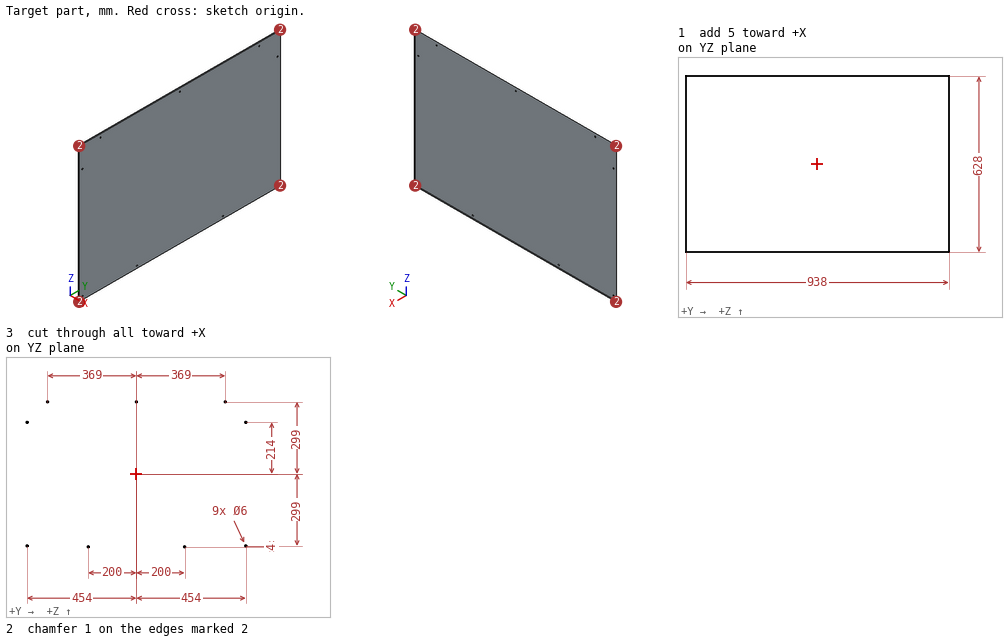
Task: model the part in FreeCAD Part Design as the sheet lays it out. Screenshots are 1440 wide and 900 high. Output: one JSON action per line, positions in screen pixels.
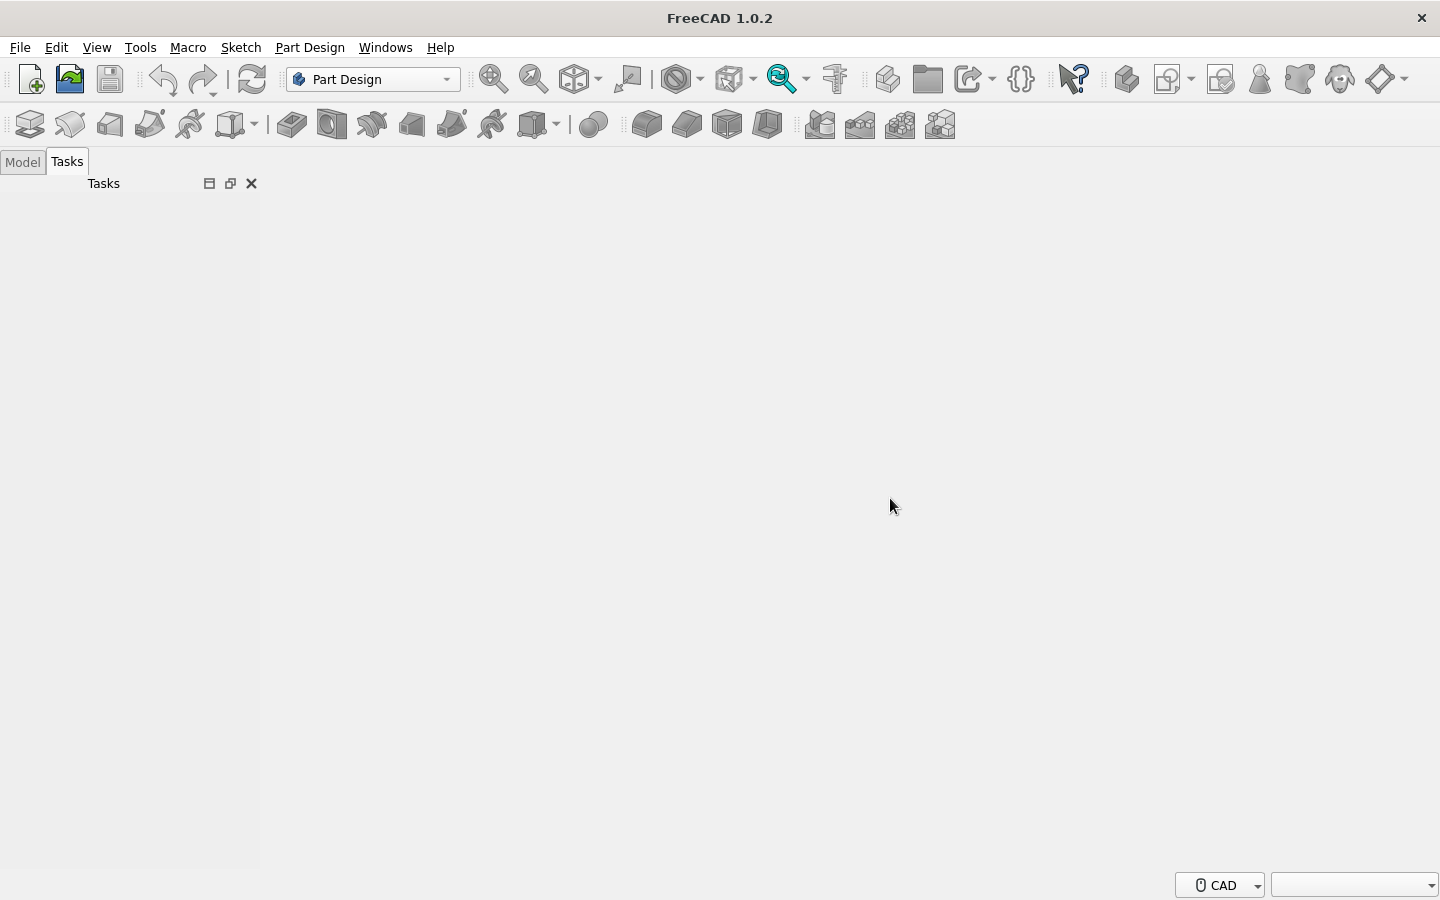
{"action": "key", "text": "ctrl+n"}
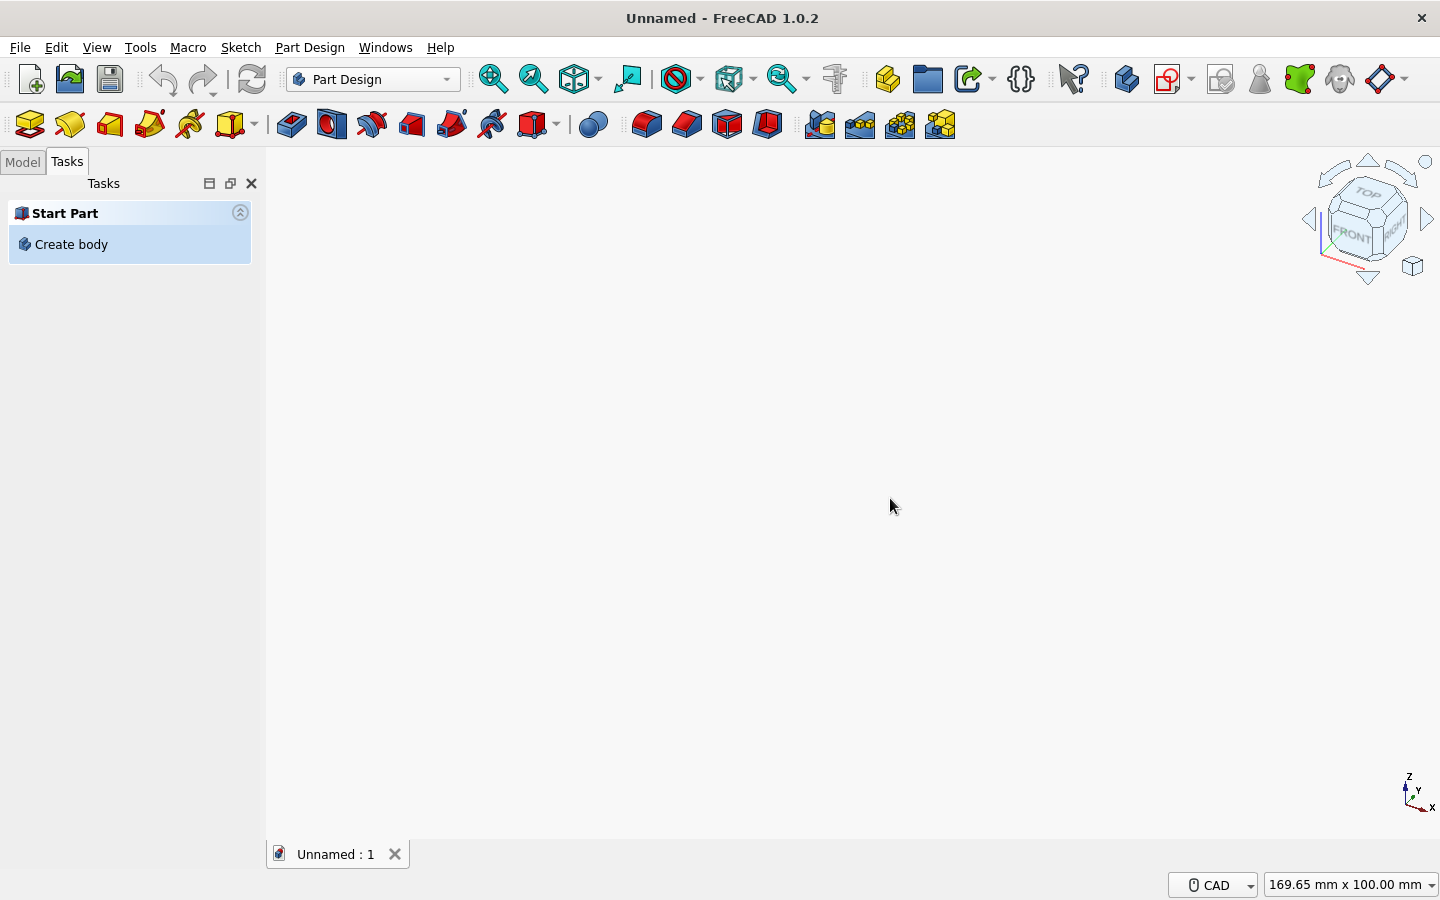
{"action": "left_click", "coordinate": [1168, 80]}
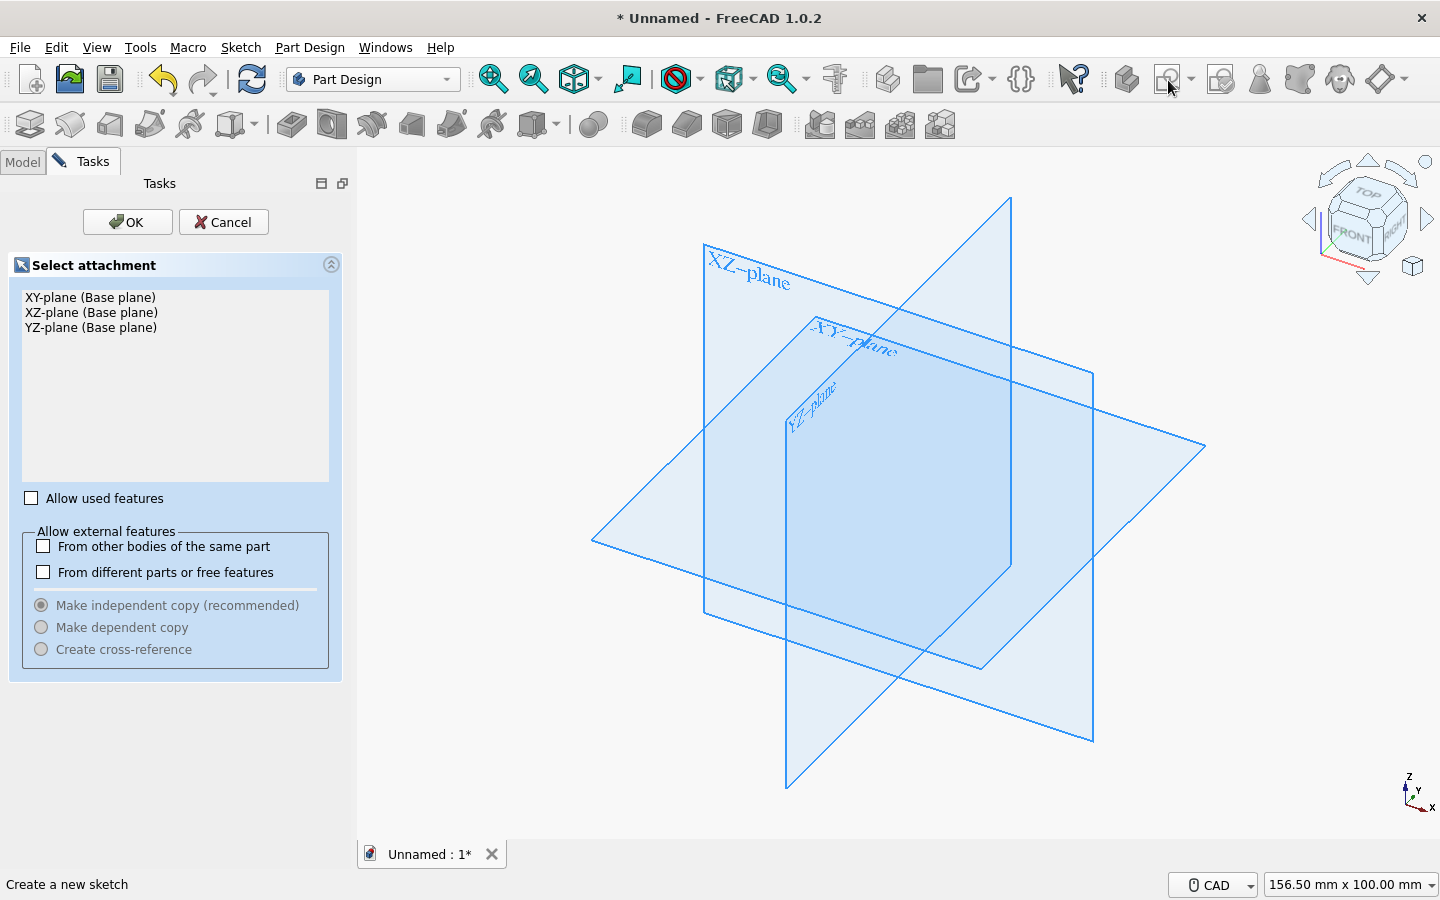
{"action": "left_click", "coordinate": [82, 328]}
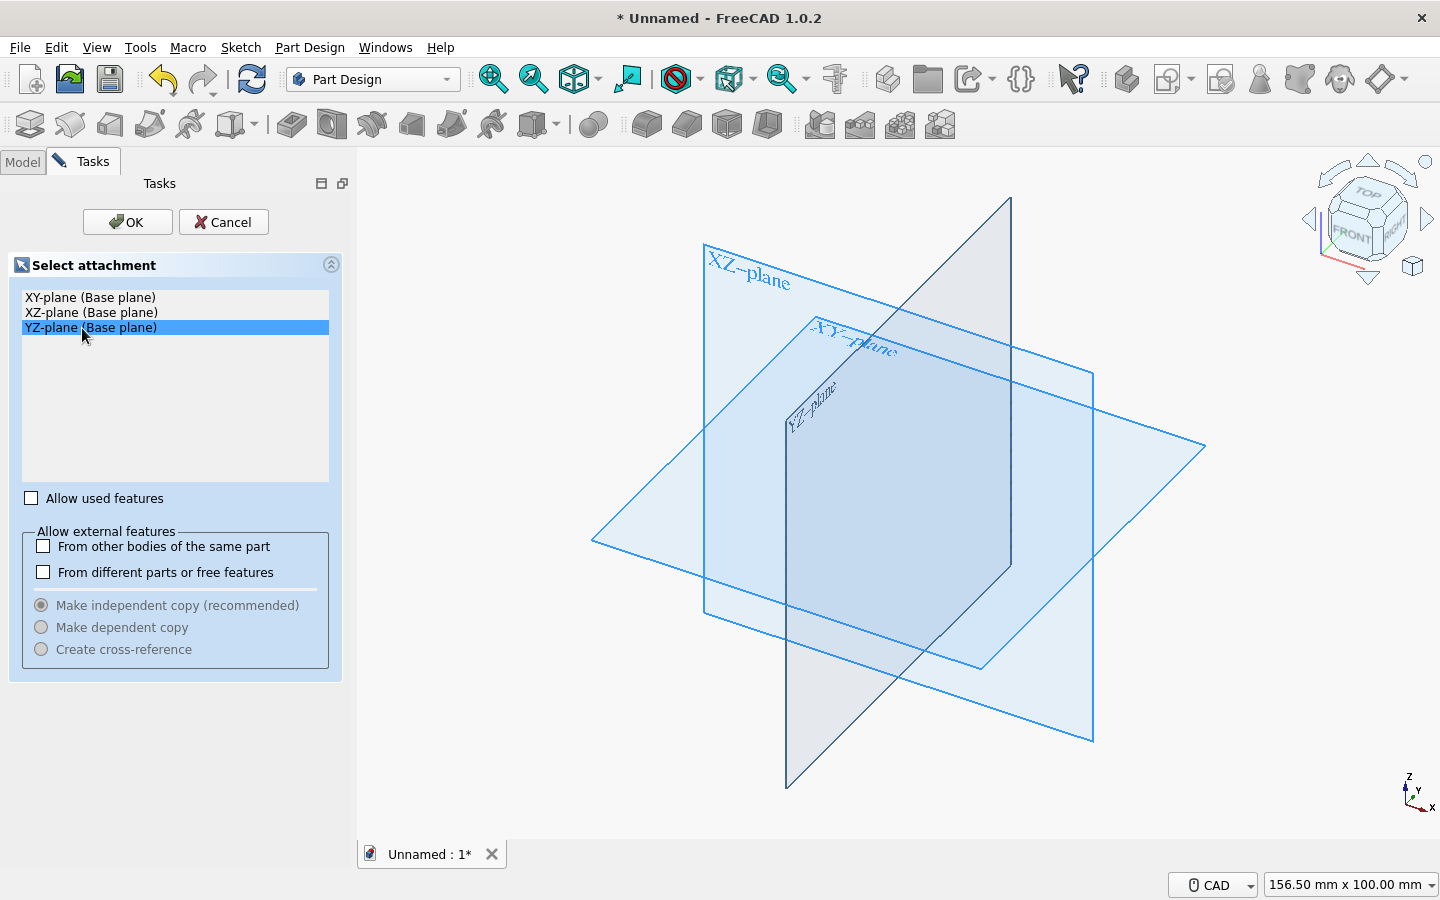
{"action": "left_click", "coordinate": [128, 222]}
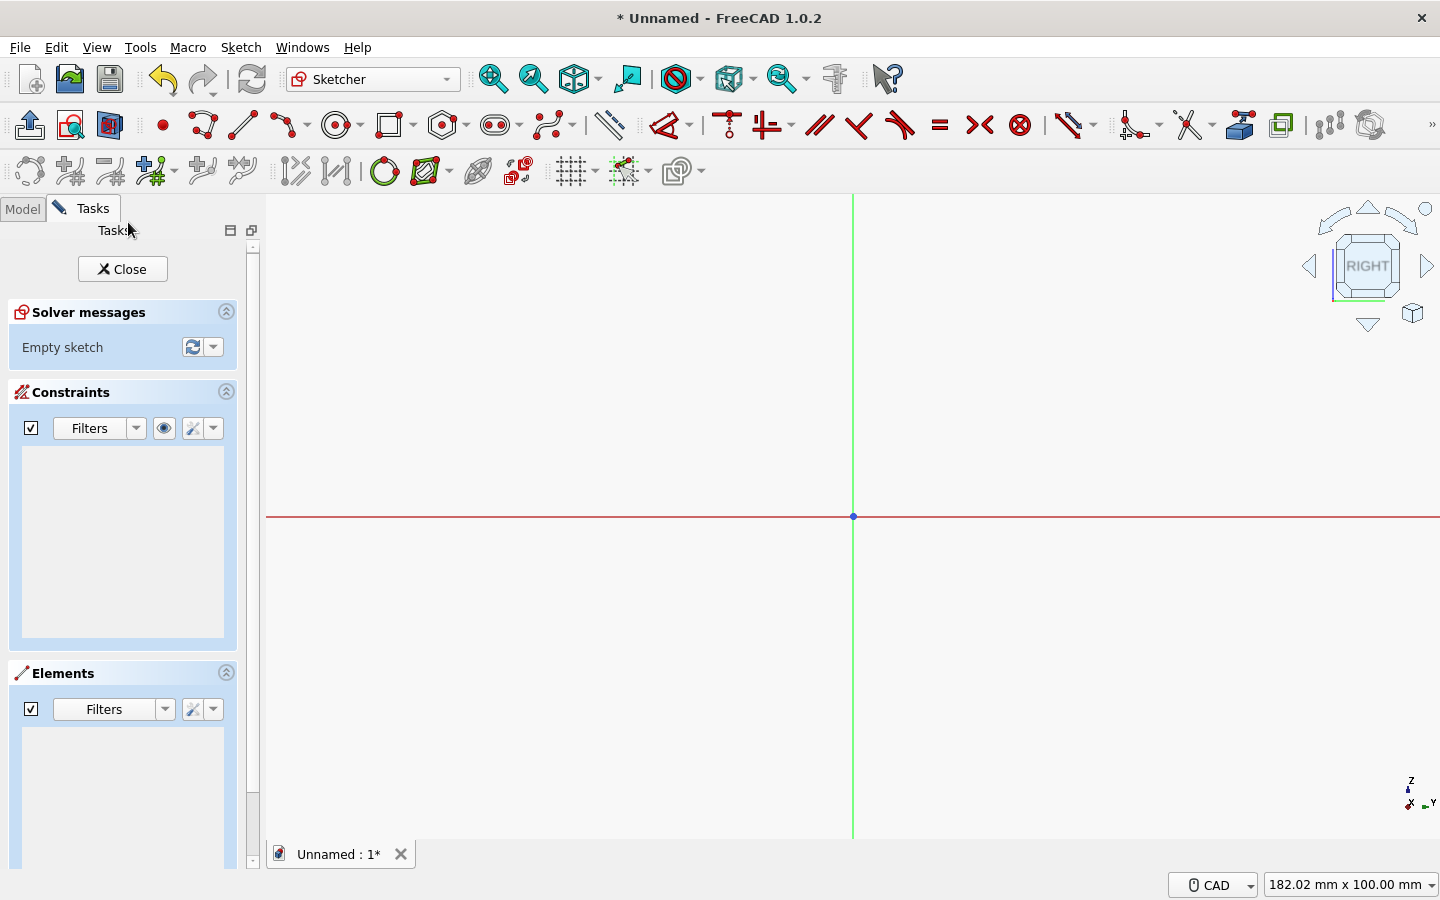
{"action": "scroll", "coordinate": [776, 516], "scroll_direction": "down", "scroll_amount": 11}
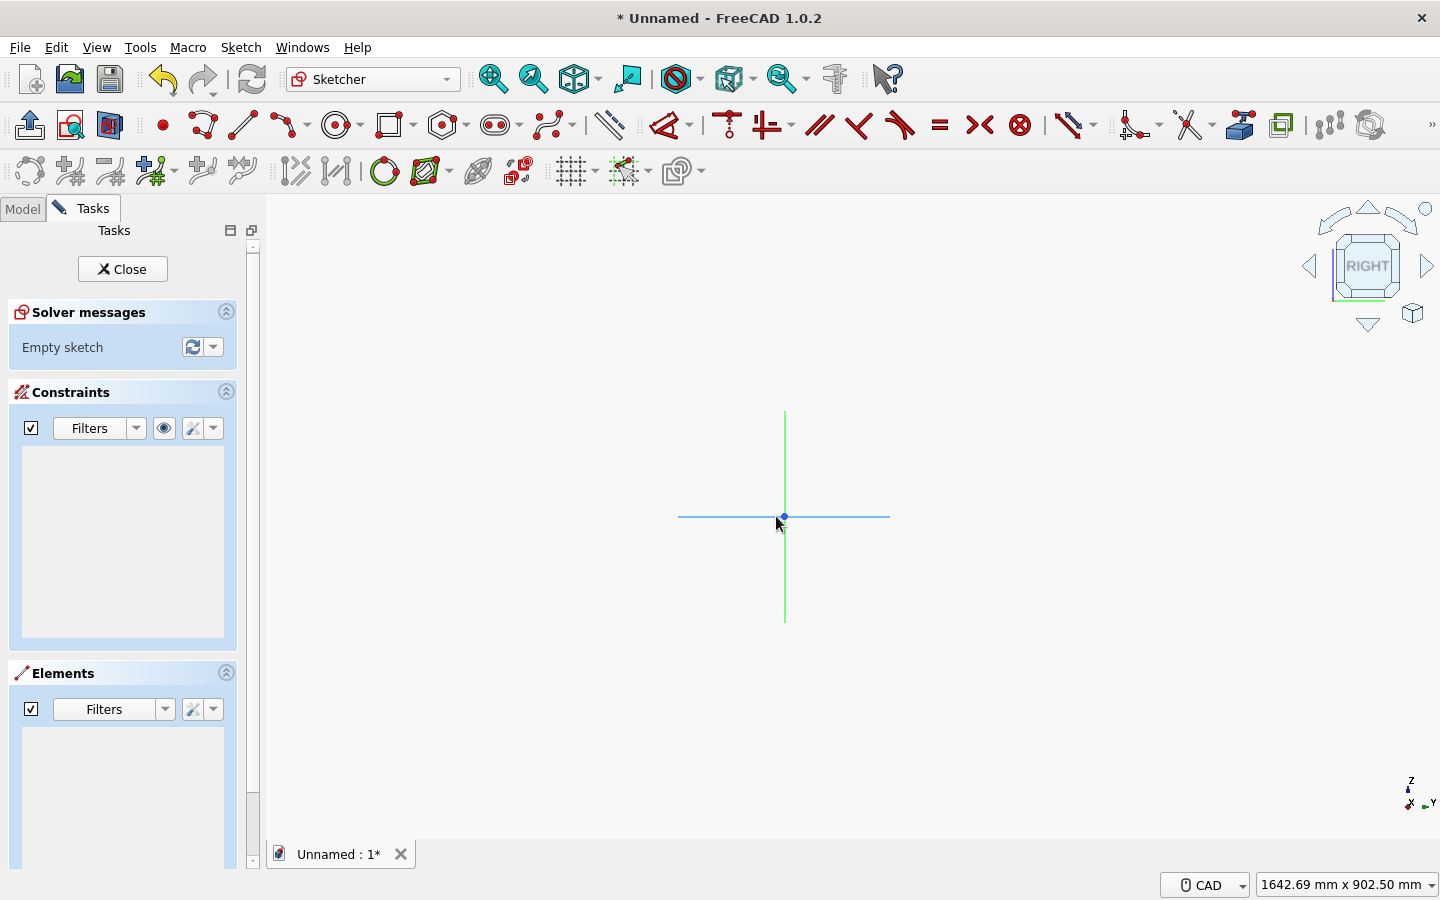
{"action": "key", "text": "g v"}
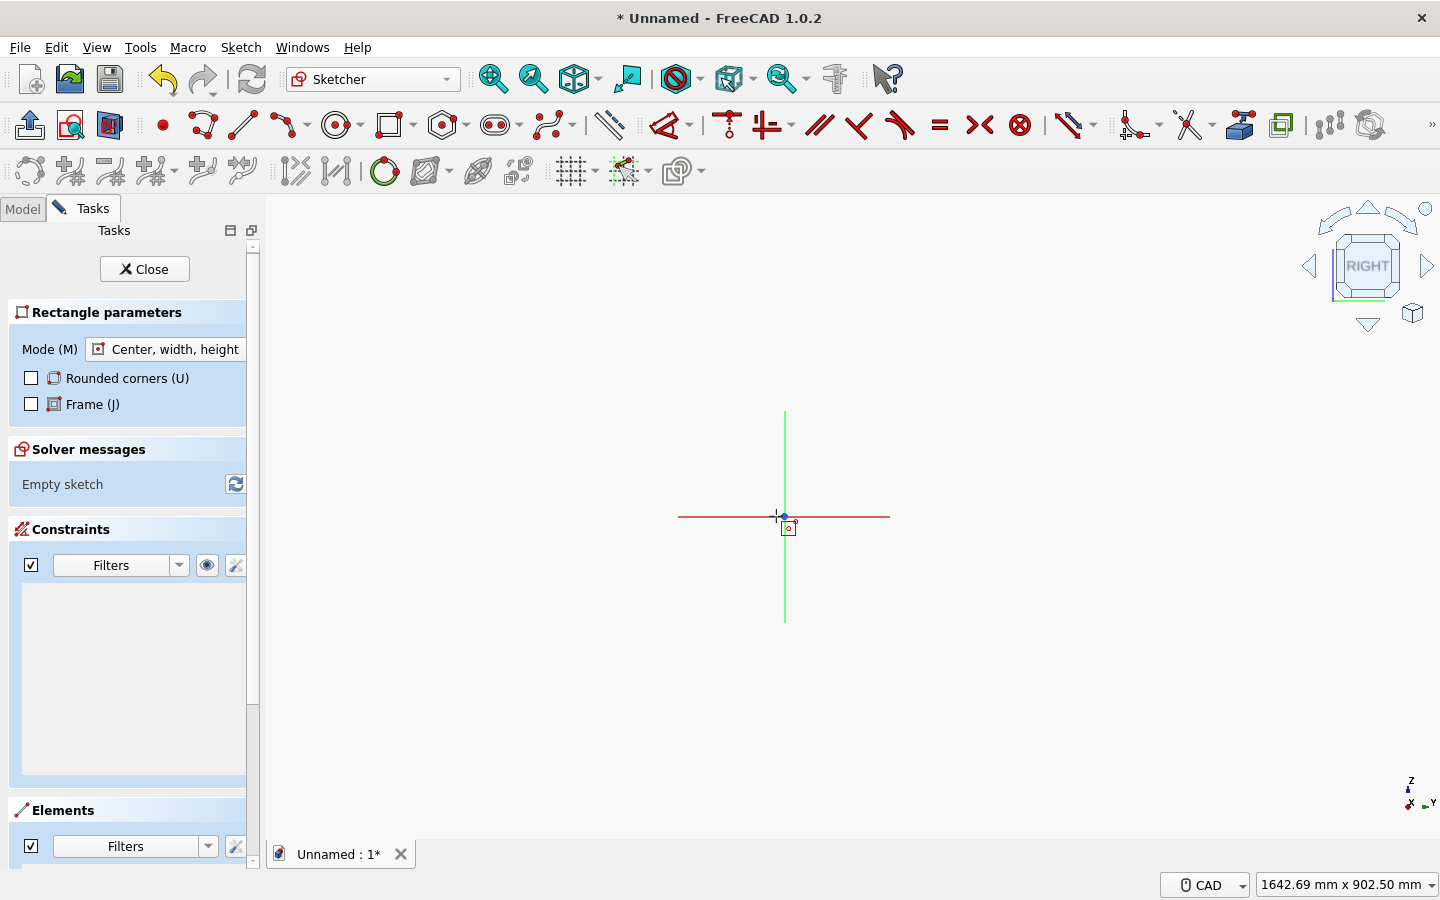
{"action": "left_click", "coordinate": [785, 516]}
{"action": "left_click", "coordinate": [1120, 292]}
{"action": "key", "text": "Escape"}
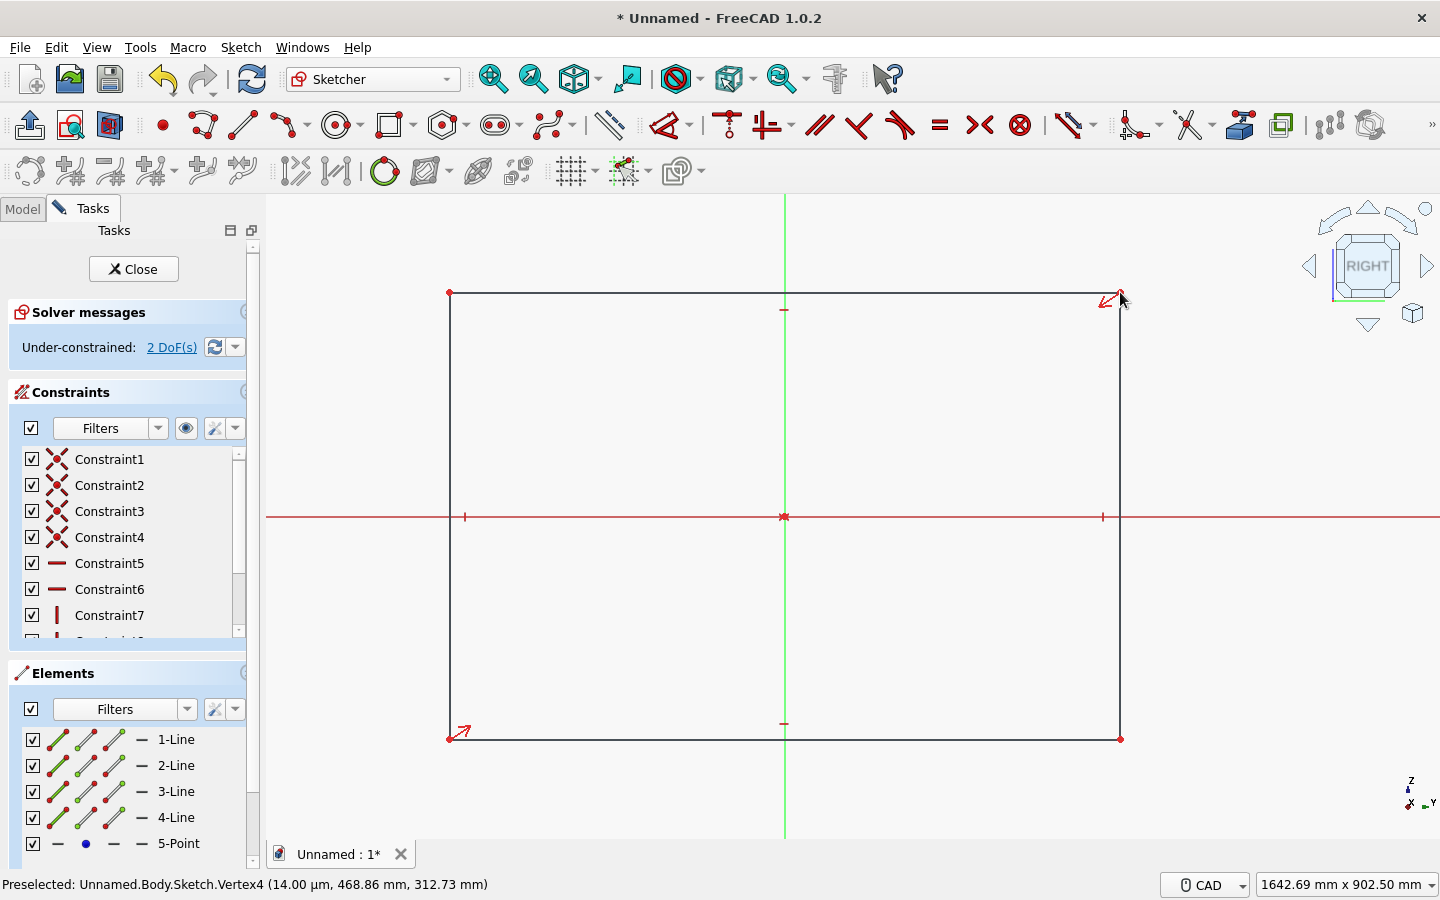
{"action": "key", "text": "d"}